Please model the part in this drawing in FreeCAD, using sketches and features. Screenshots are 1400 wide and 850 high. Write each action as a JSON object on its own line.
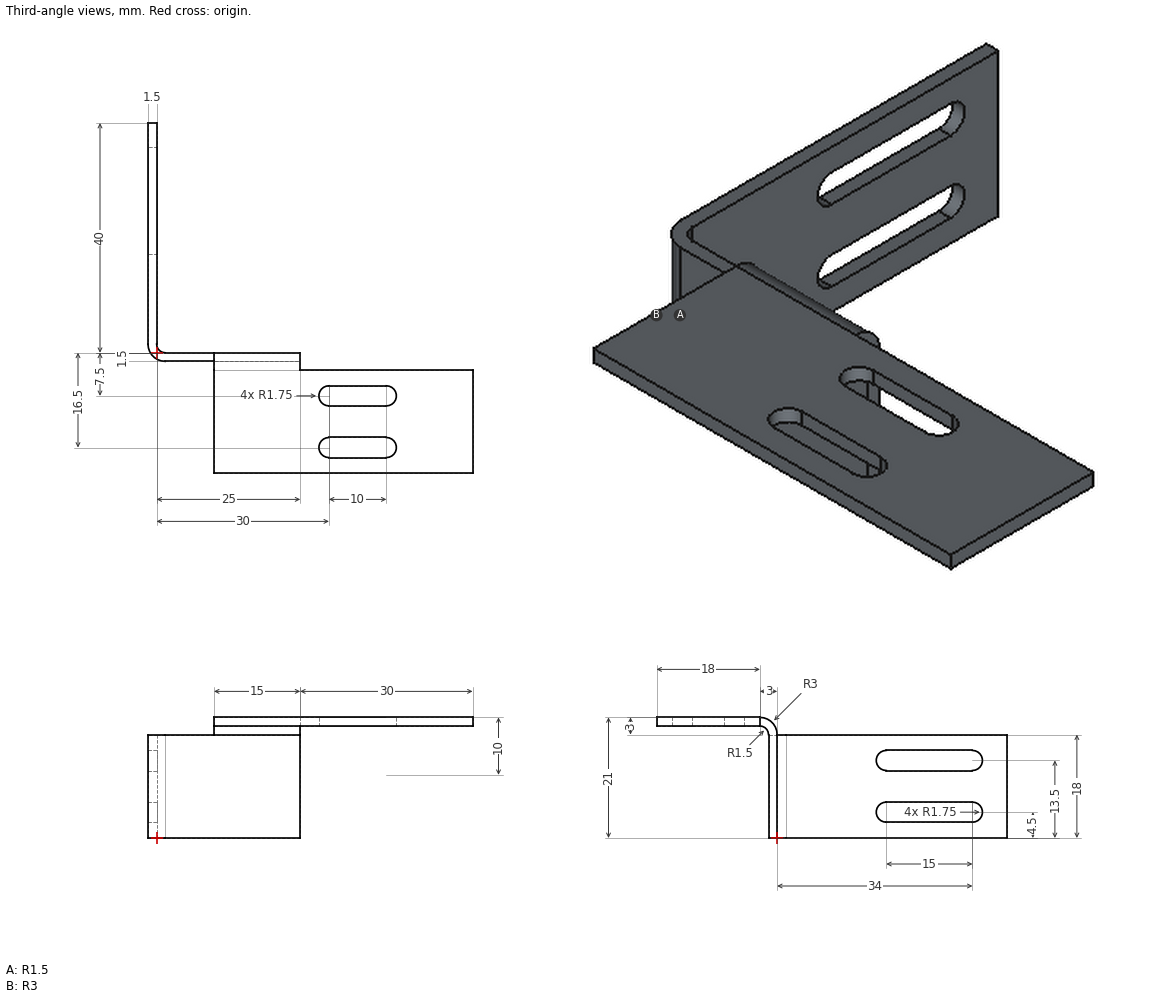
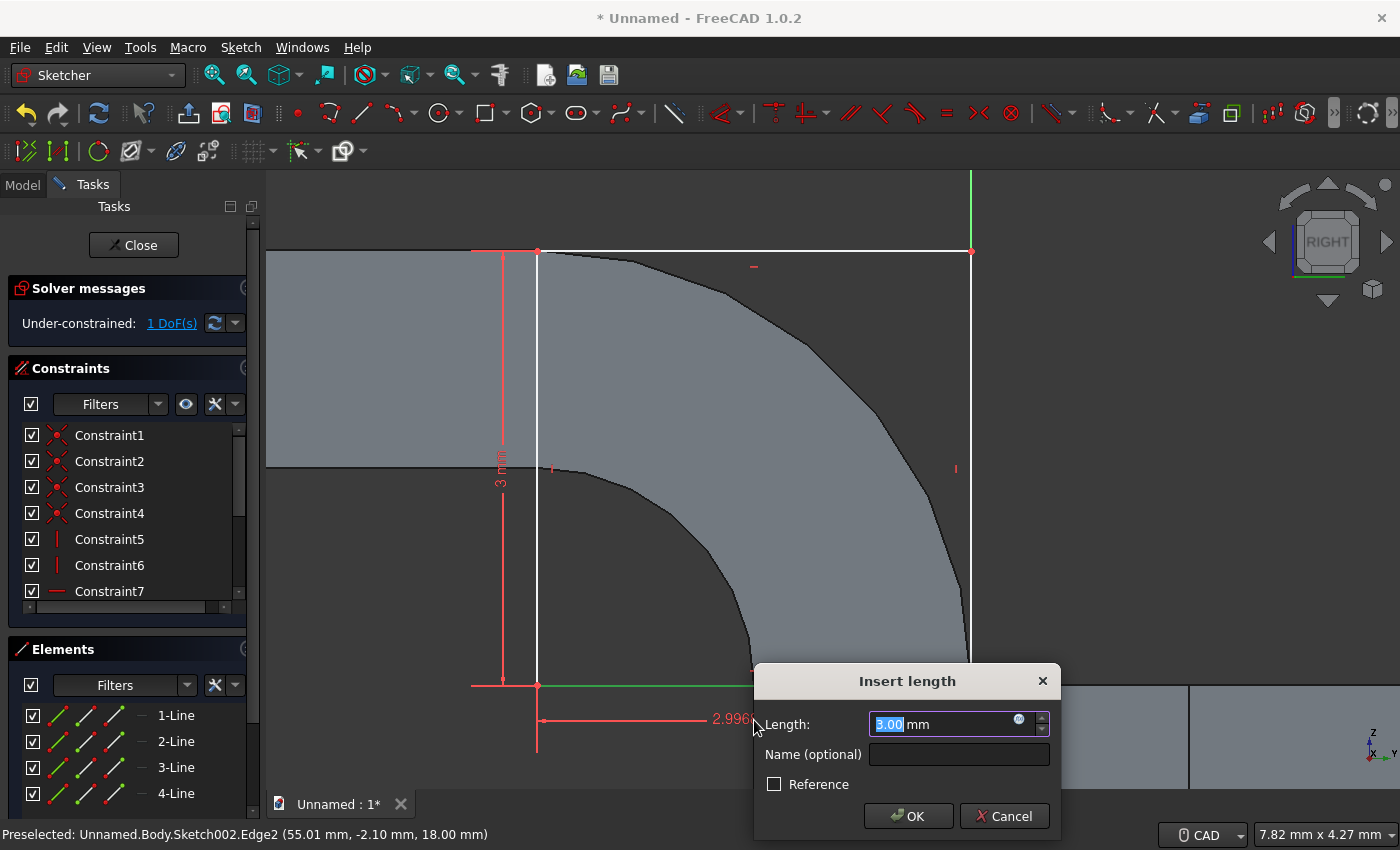
{"action": "type", "text": "3"}
{"action": "key", "text": "Return"}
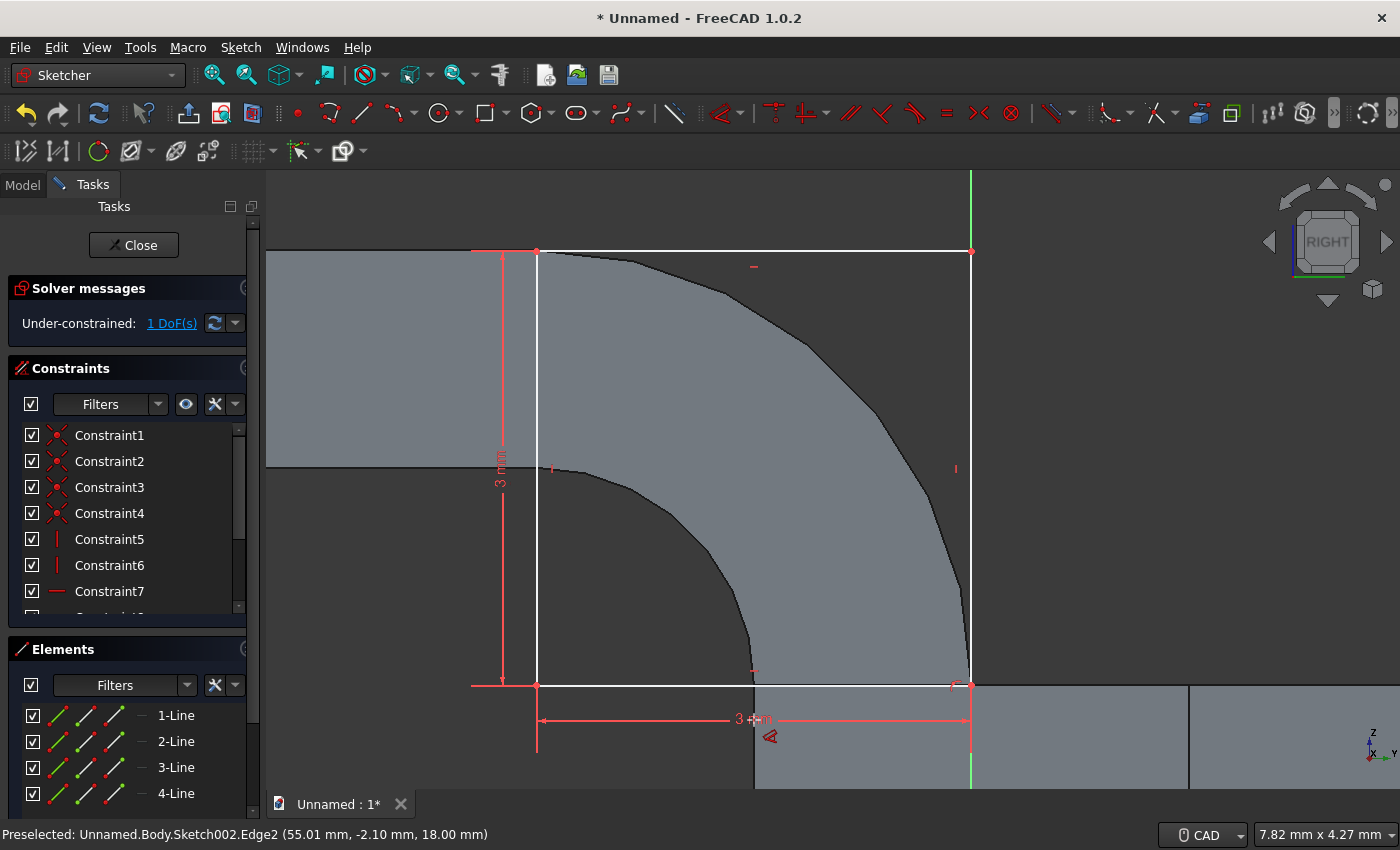
{"action": "left_click", "coordinate": [537, 251]}
{"action": "left_click", "coordinate": [1005, 506]}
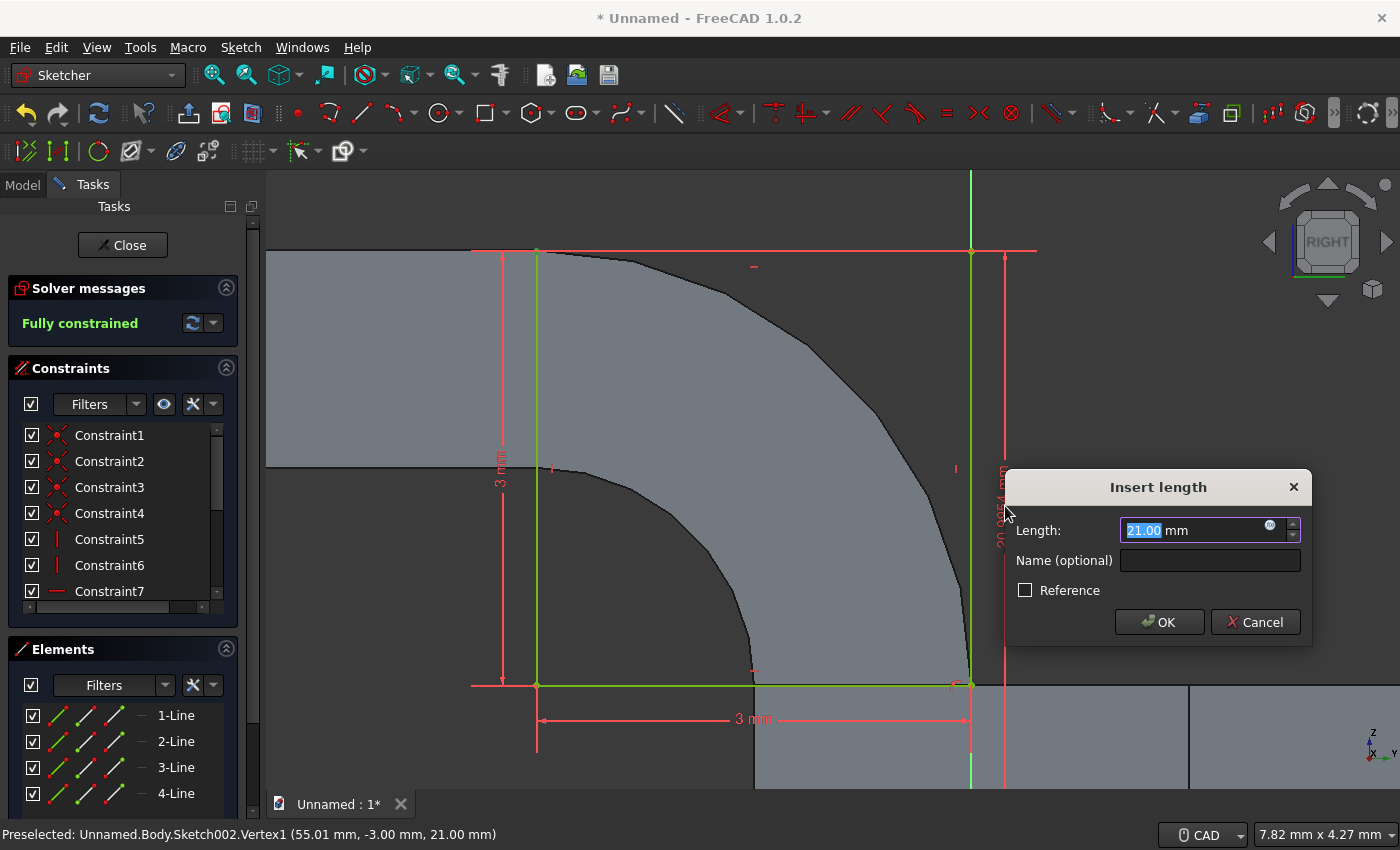
{"action": "type", "text": "21"}
{"action": "key", "text": "Return"}
{"action": "key", "text": "Escape"}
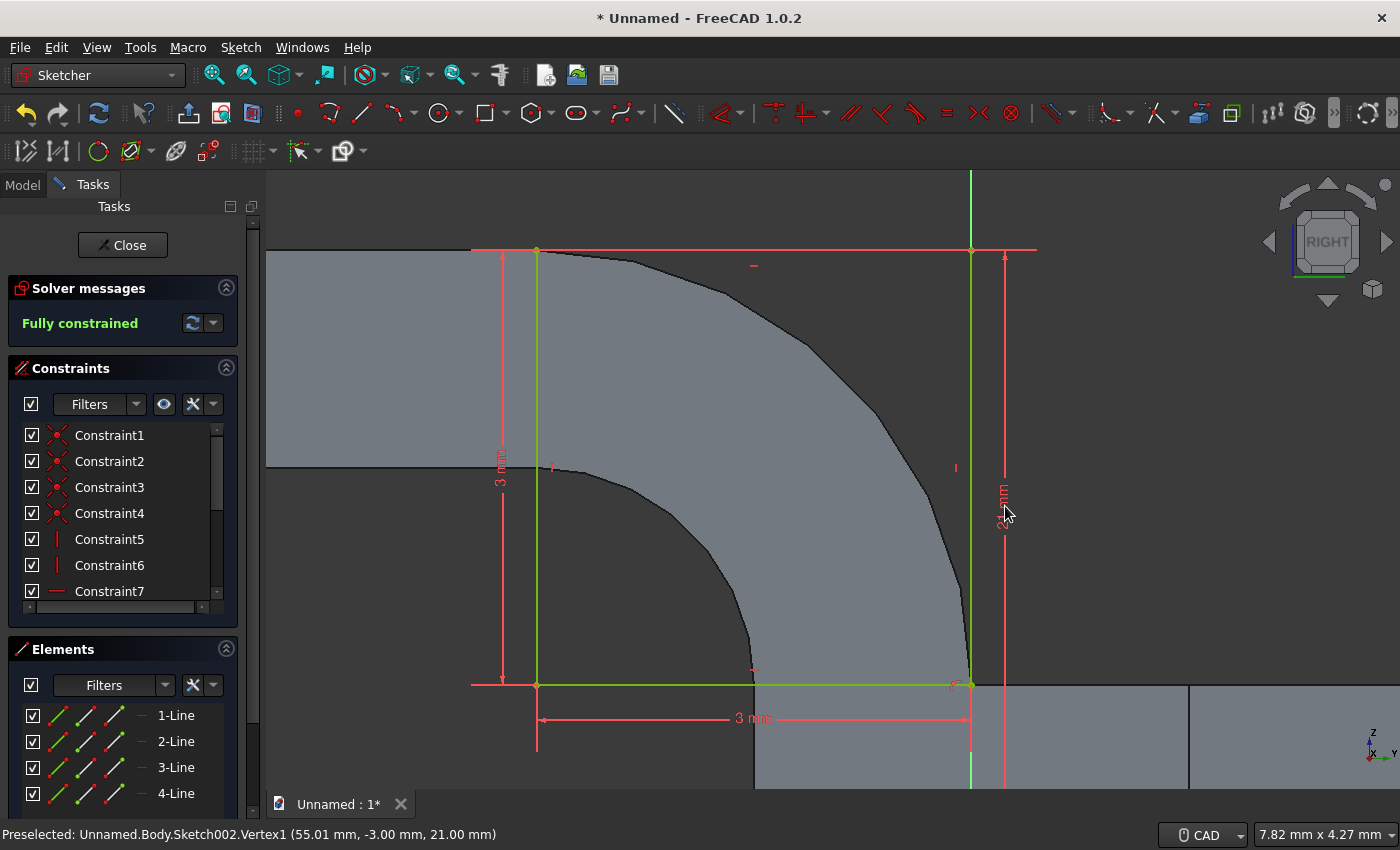
{"action": "left_click", "coordinate": [123, 245]}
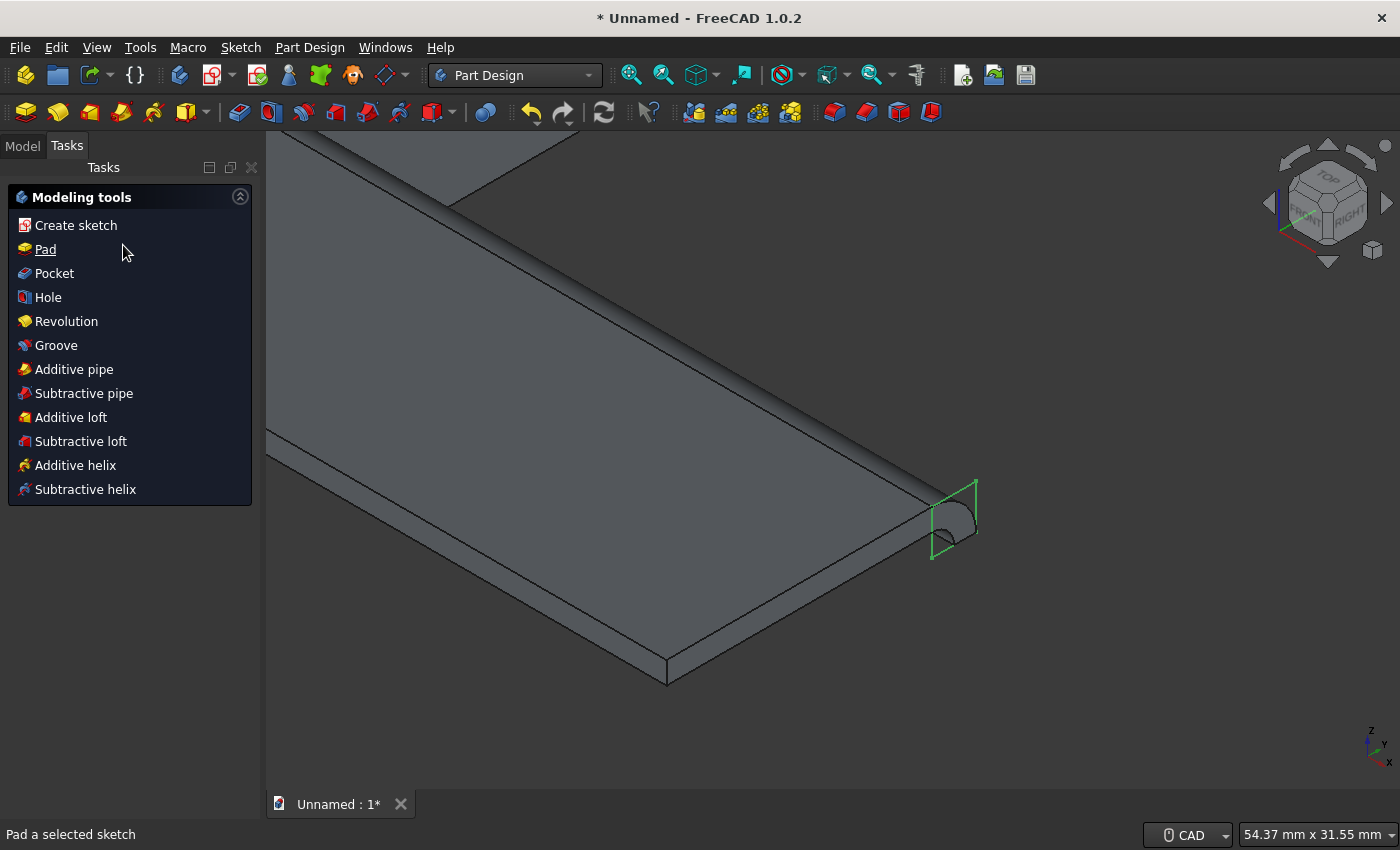
{"action": "left_click", "coordinate": [240, 112]}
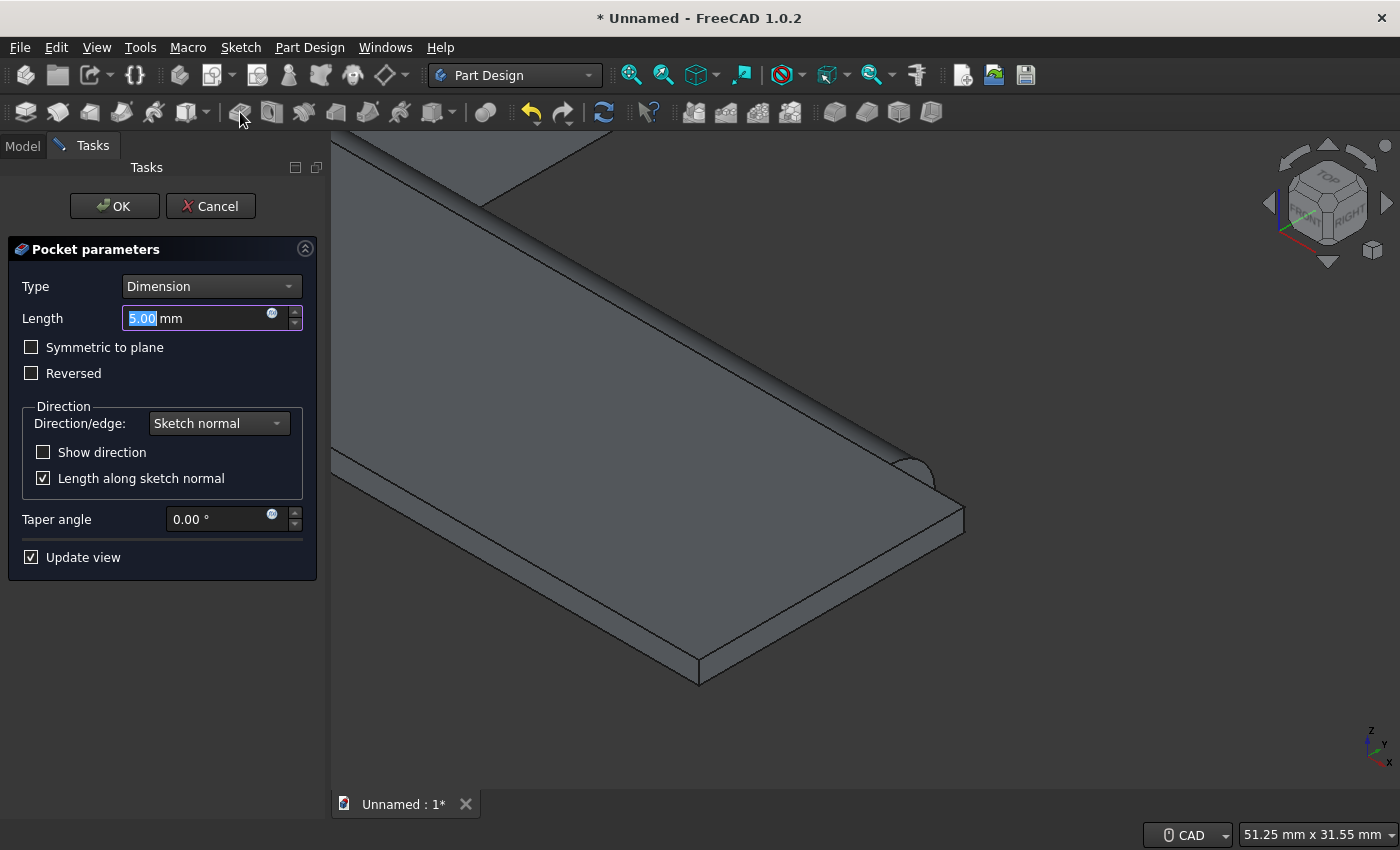
{"action": "type", "text": "30"}
{"action": "key", "text": "Tab"}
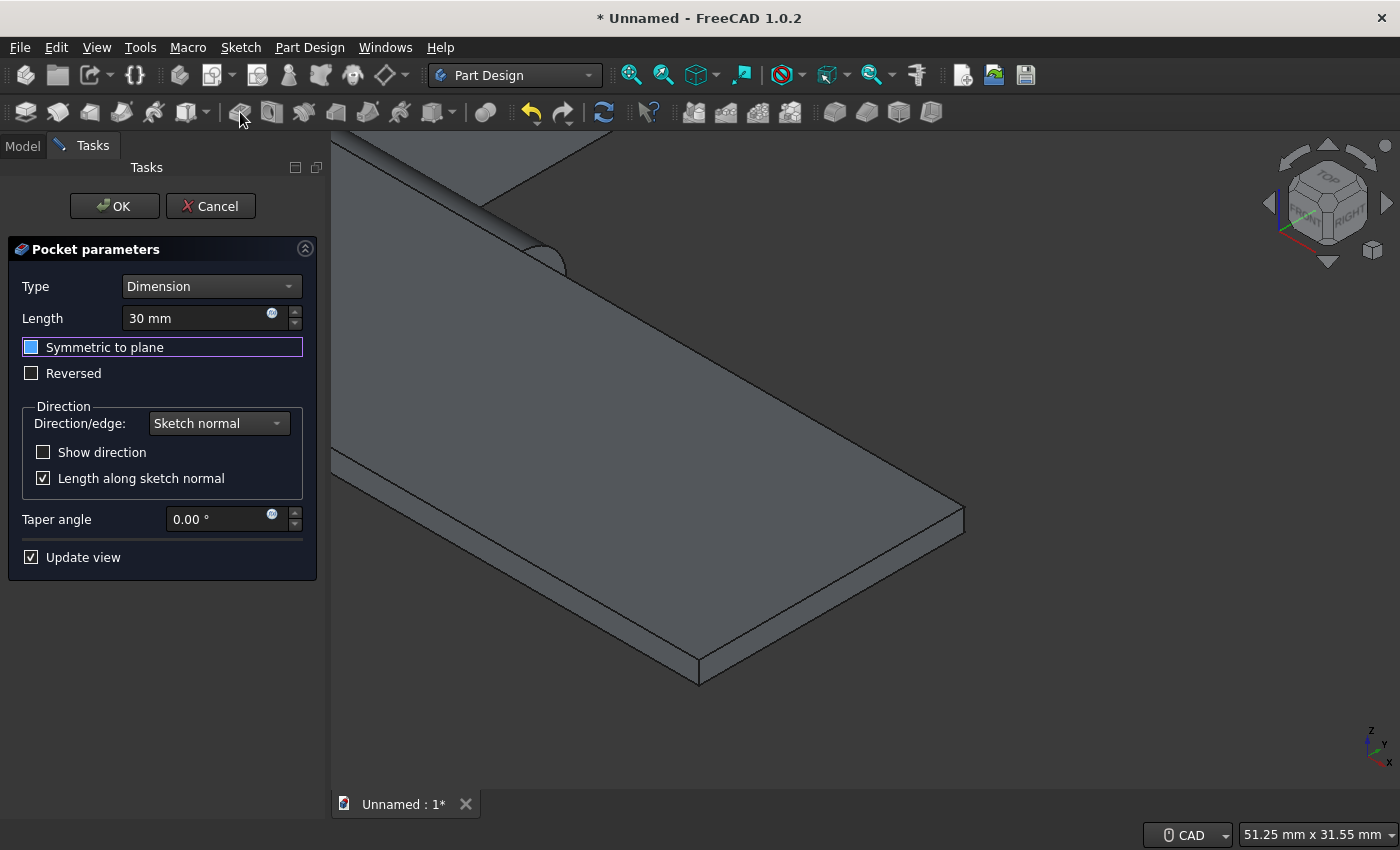
{"action": "left_click", "coordinate": [115, 206]}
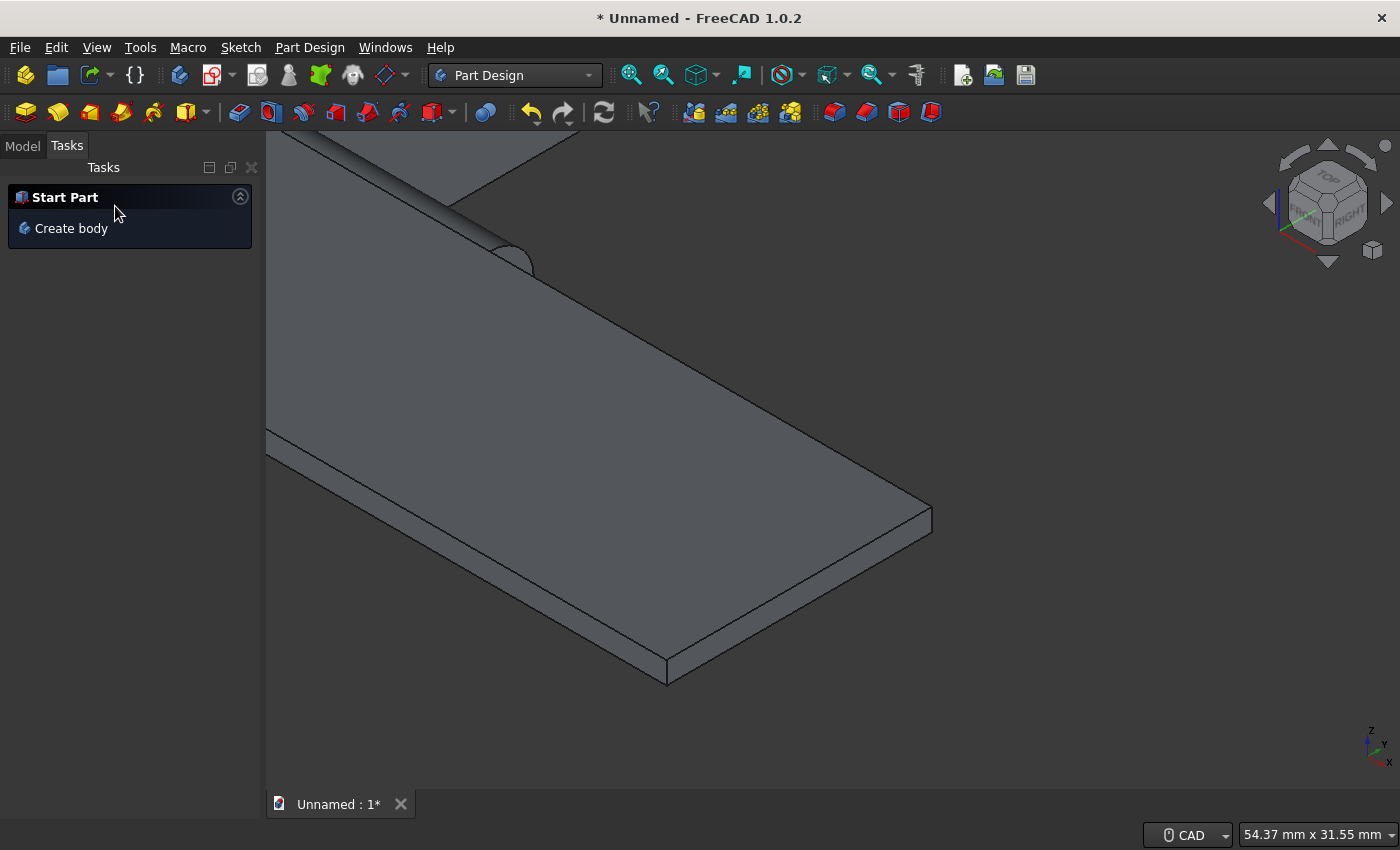
{"action": "key", "text": "v f"}